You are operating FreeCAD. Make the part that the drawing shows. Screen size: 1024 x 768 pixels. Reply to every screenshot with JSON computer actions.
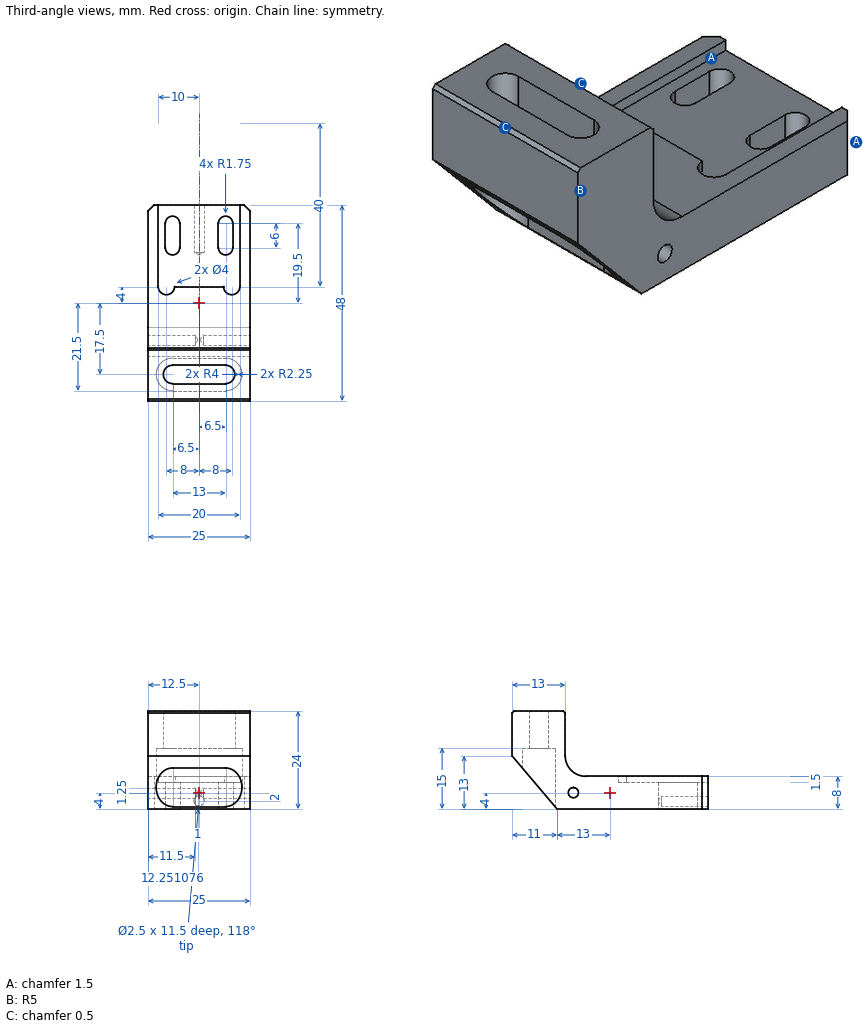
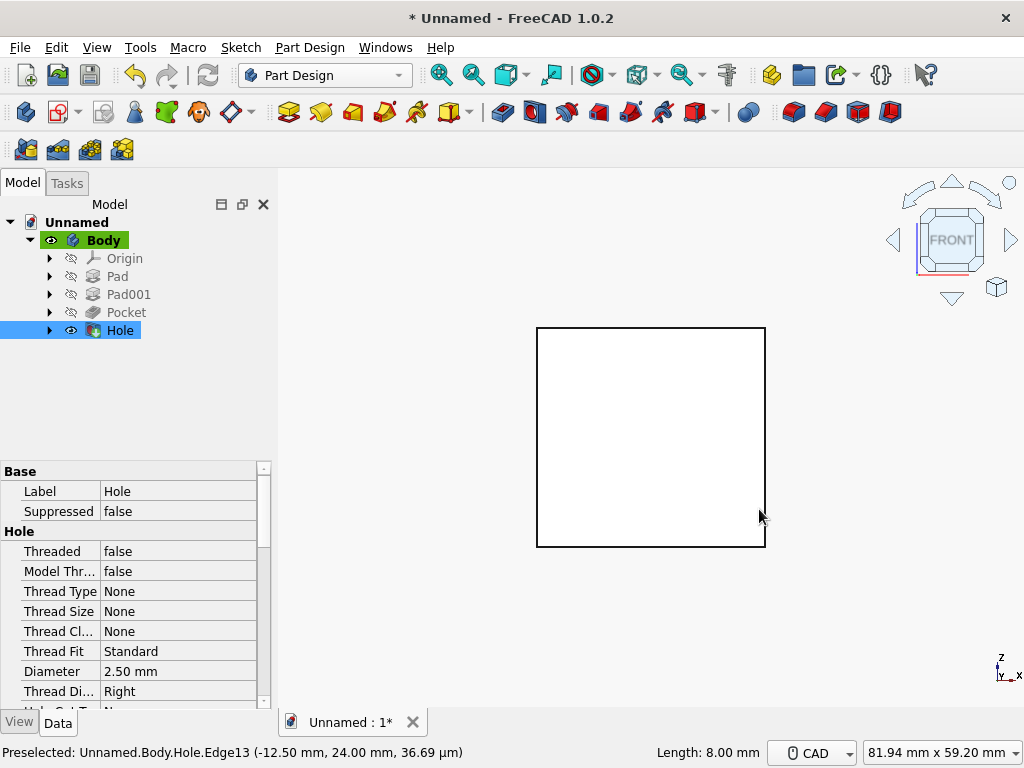
{"action": "left_click", "coordinate": [442, 76]}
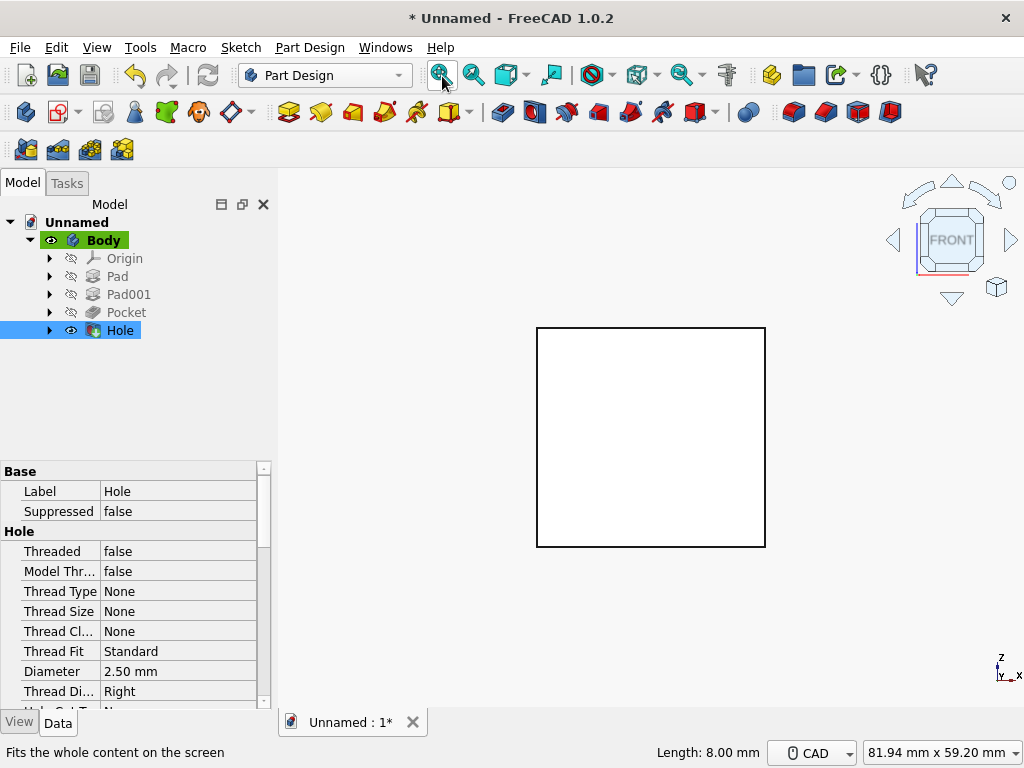
{"action": "key", "text": "3"}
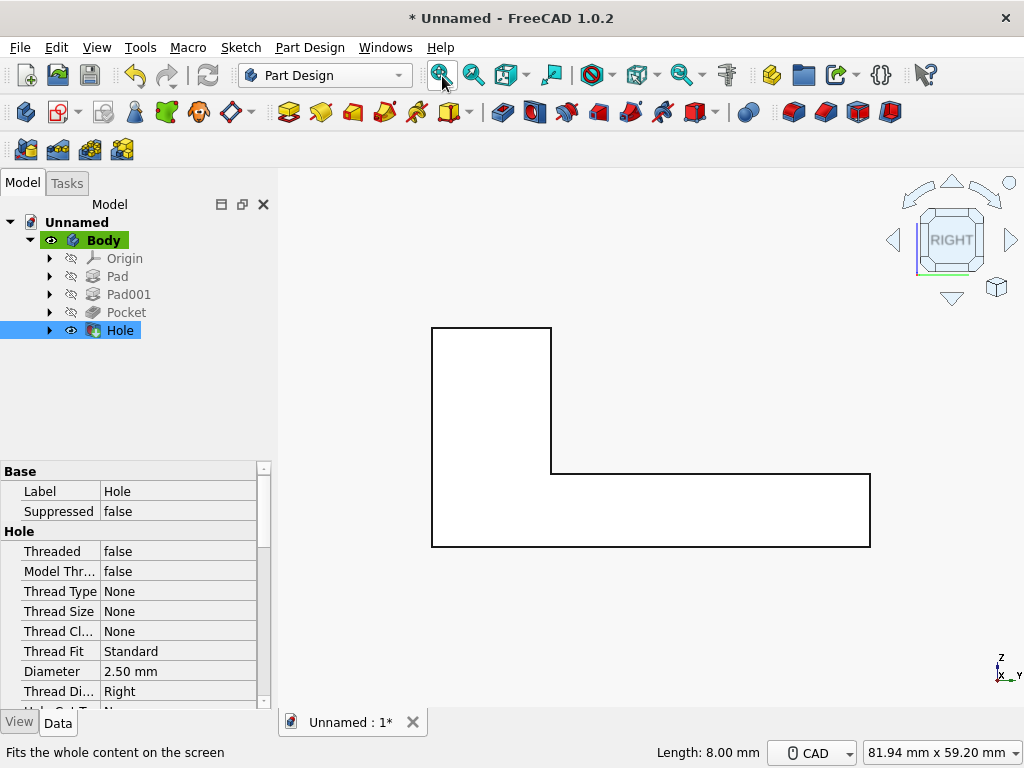
{"action": "left_click", "coordinate": [870, 509], "text": "ctrl"}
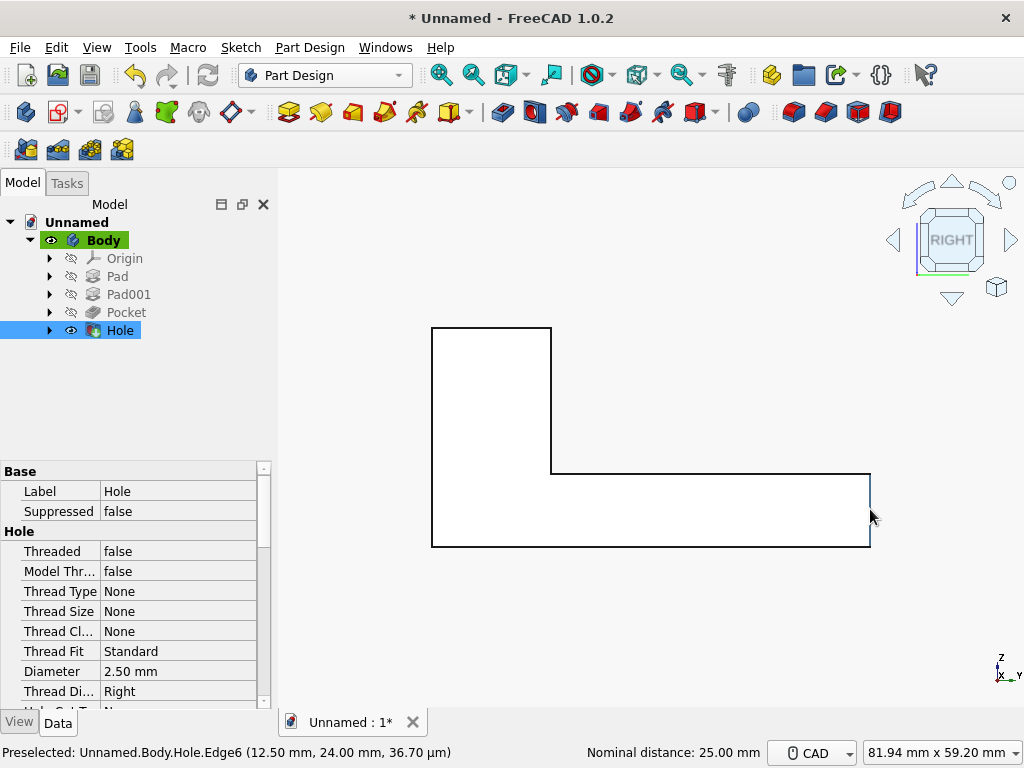
{"action": "left_click", "coordinate": [826, 112]}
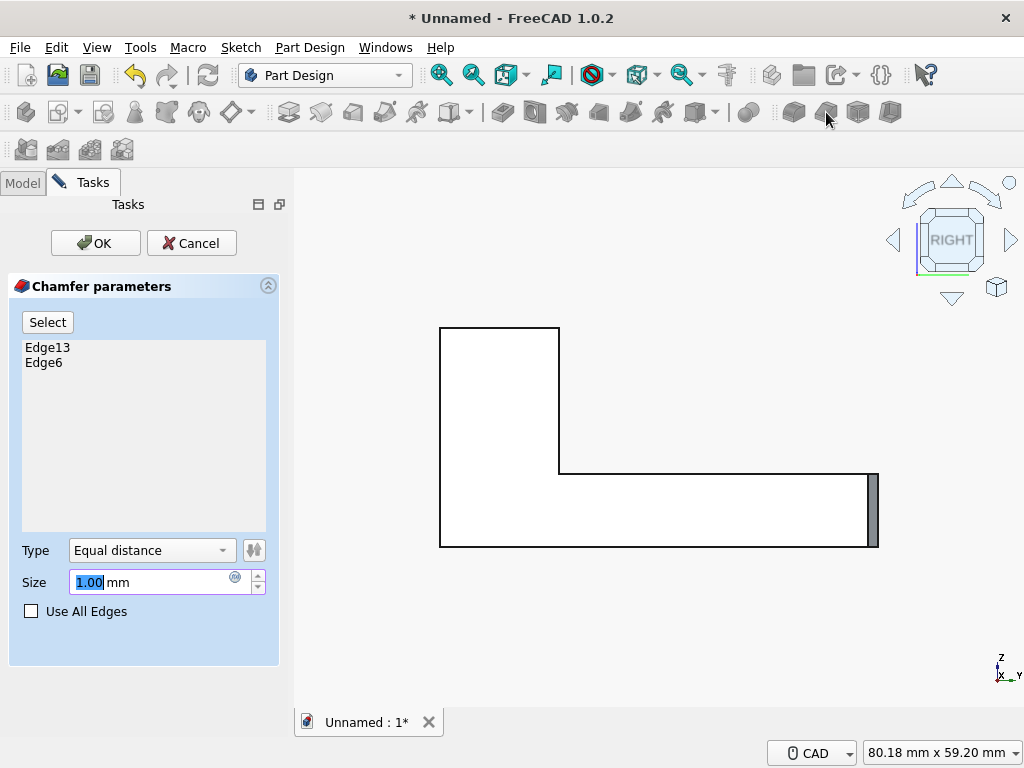
{"action": "type", "text": "1.5"}
{"action": "key", "text": "Tab"}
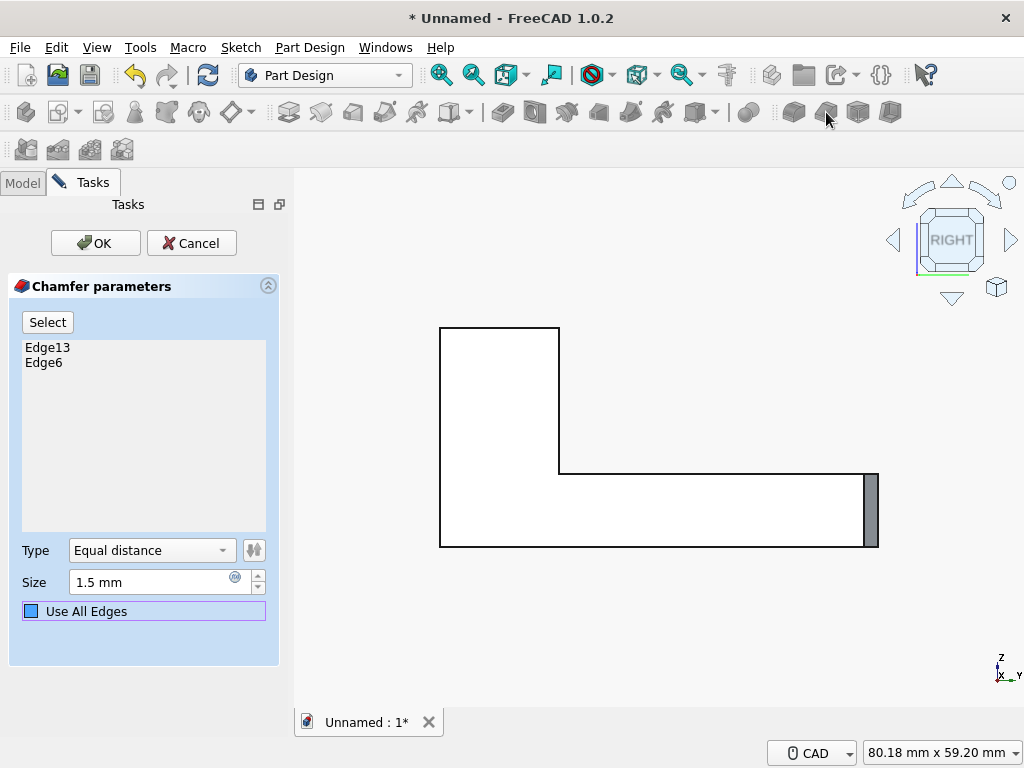
{"action": "left_click", "coordinate": [96, 243]}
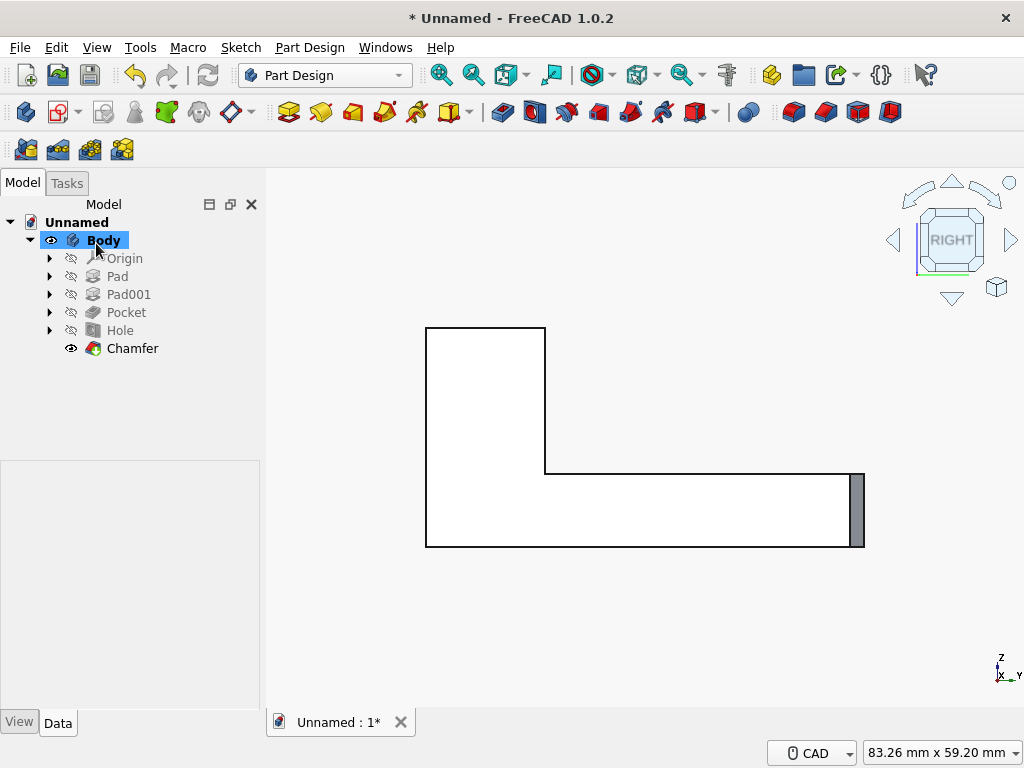
{"action": "key", "text": "5"}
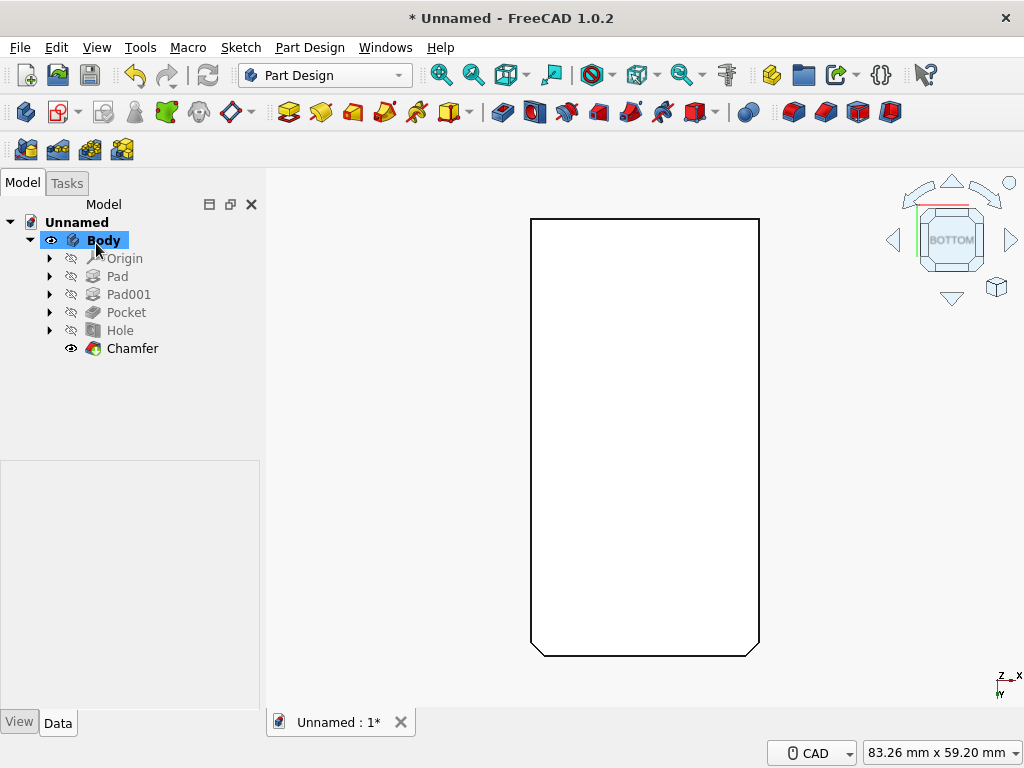
{"action": "left_click", "coordinate": [645, 499]}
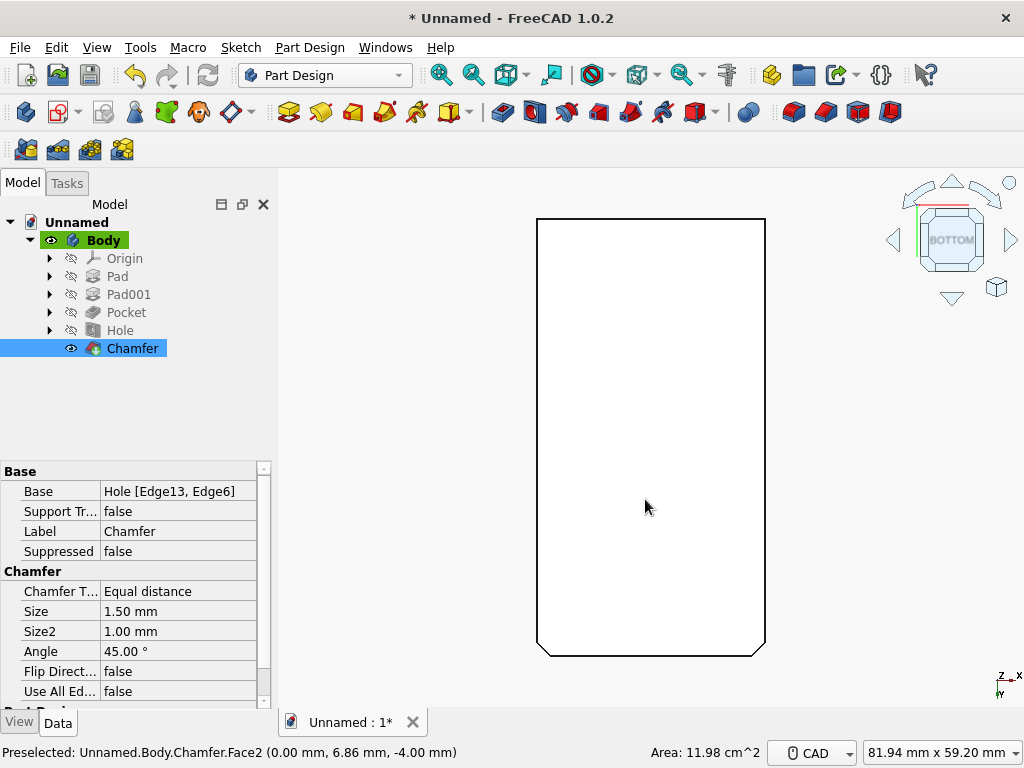
{"action": "left_click", "coordinate": [58, 112]}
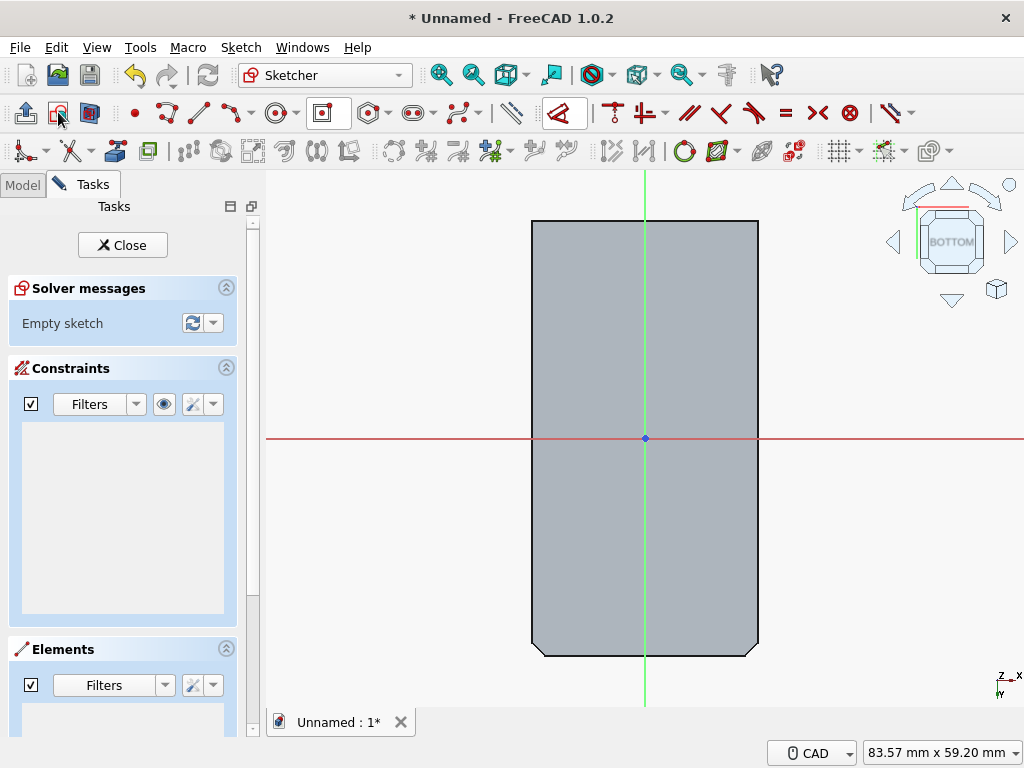
{"action": "scroll", "coordinate": [728, 652], "scroll_direction": "up", "scroll_amount": 3}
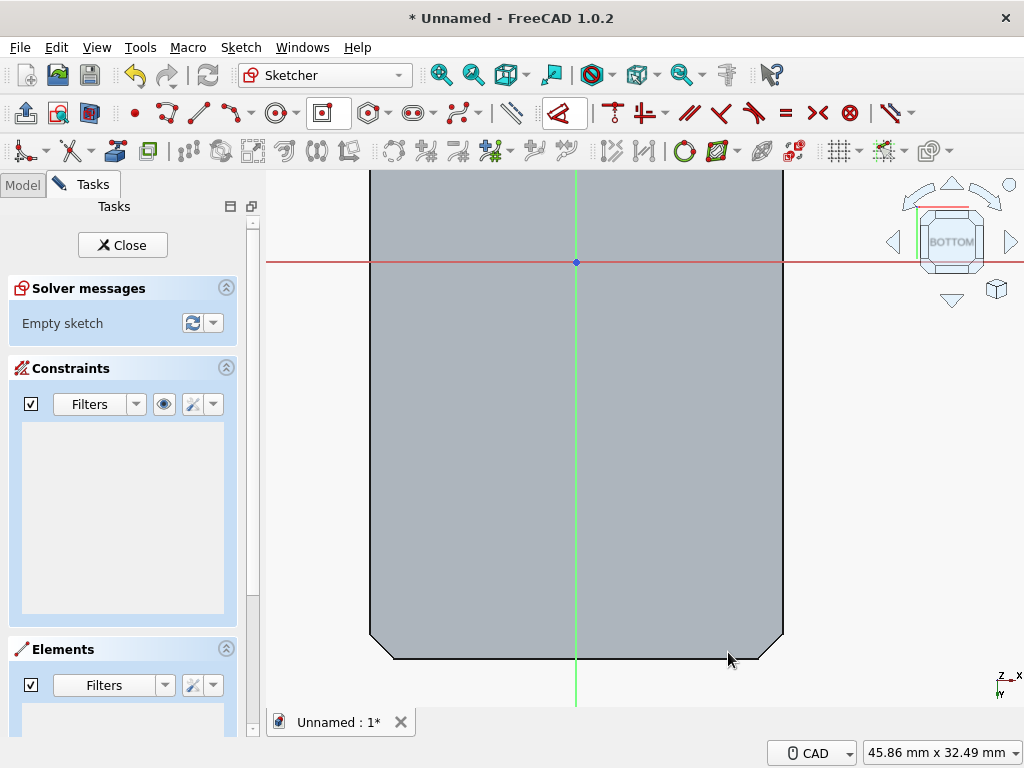
{"action": "left_click", "coordinate": [414, 114]}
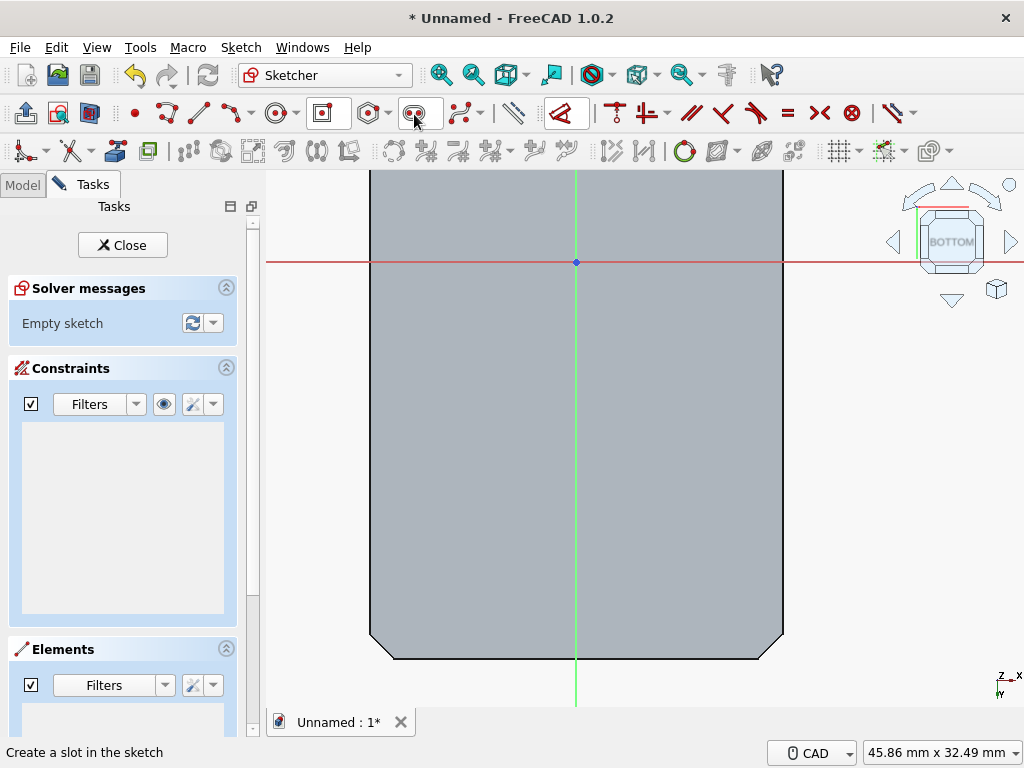
{"action": "left_click", "coordinate": [684, 585]}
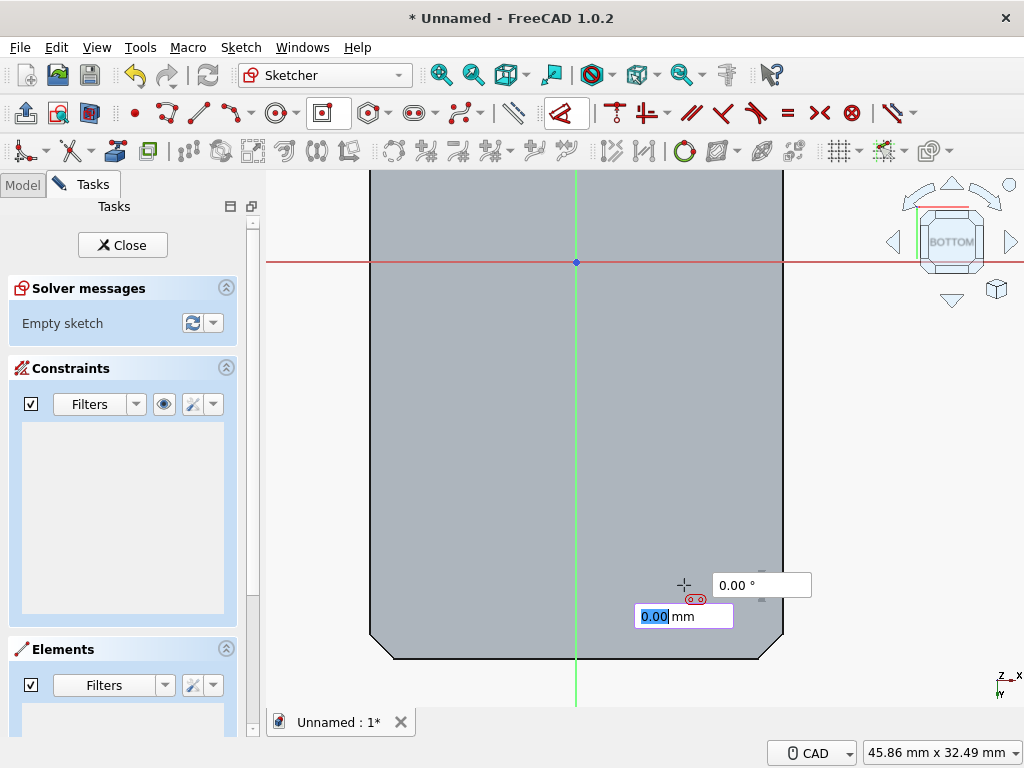
{"action": "left_click", "coordinate": [684, 485]}